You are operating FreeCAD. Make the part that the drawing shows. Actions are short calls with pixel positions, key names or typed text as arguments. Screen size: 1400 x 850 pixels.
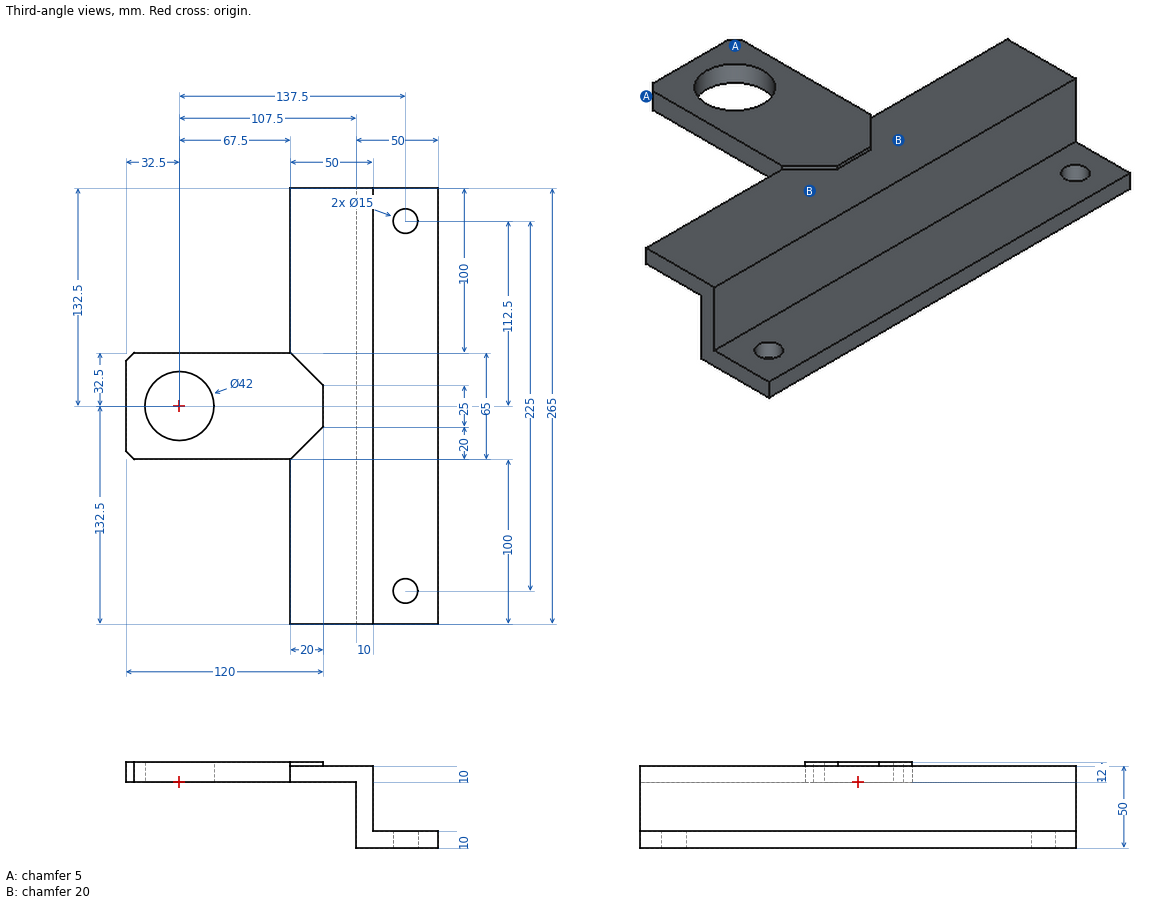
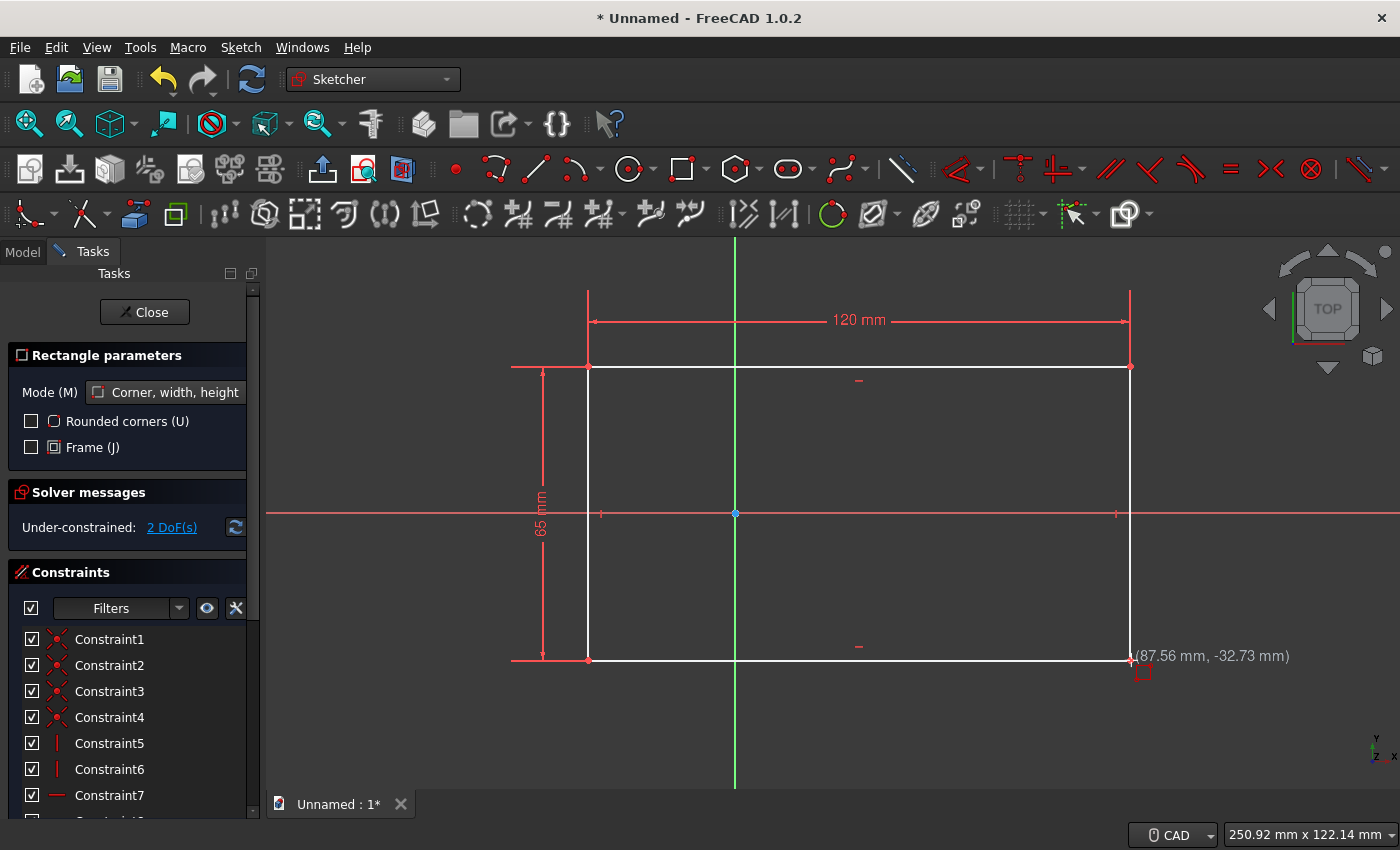
click(630, 170)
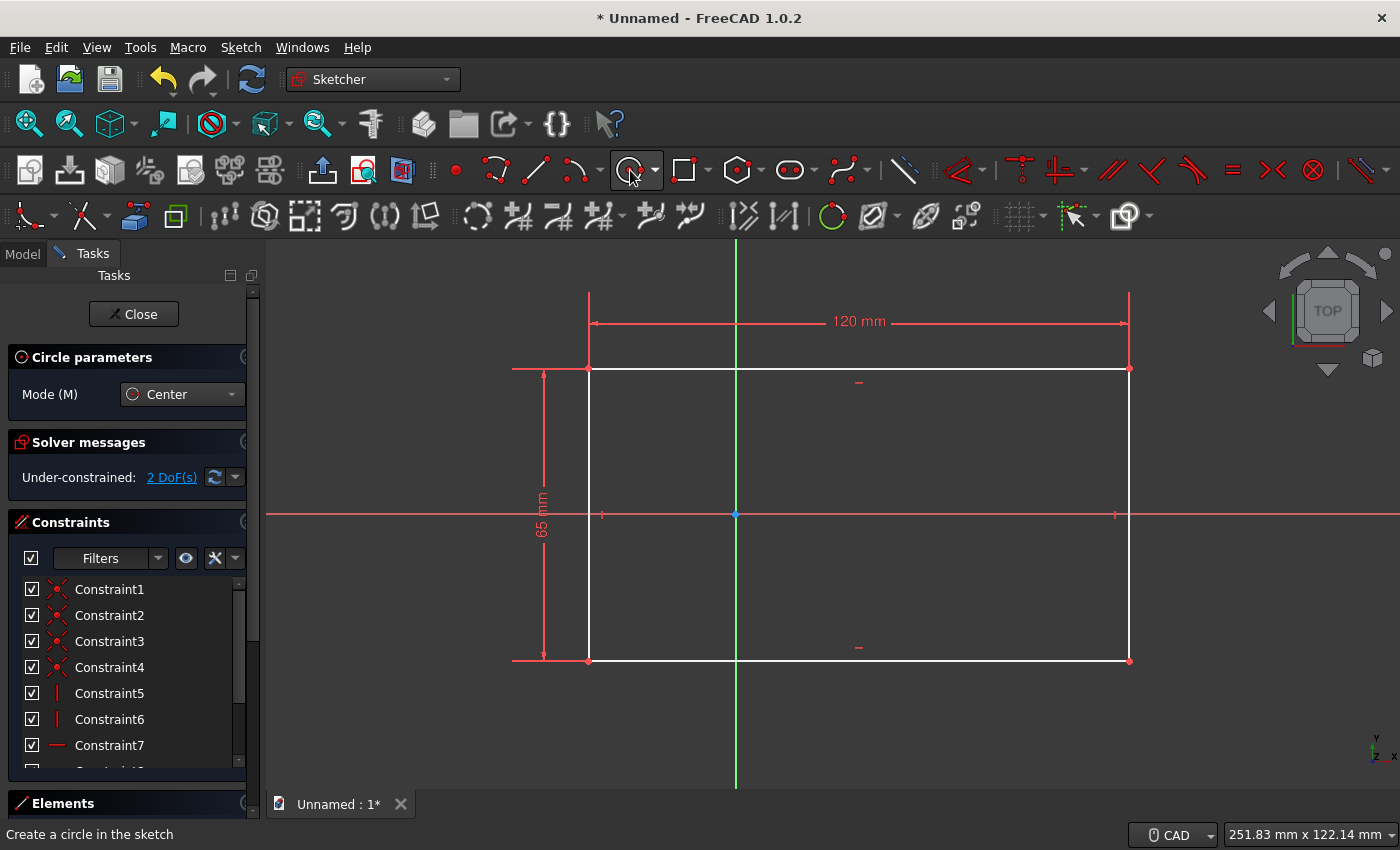
click(736, 514)
move(803, 447)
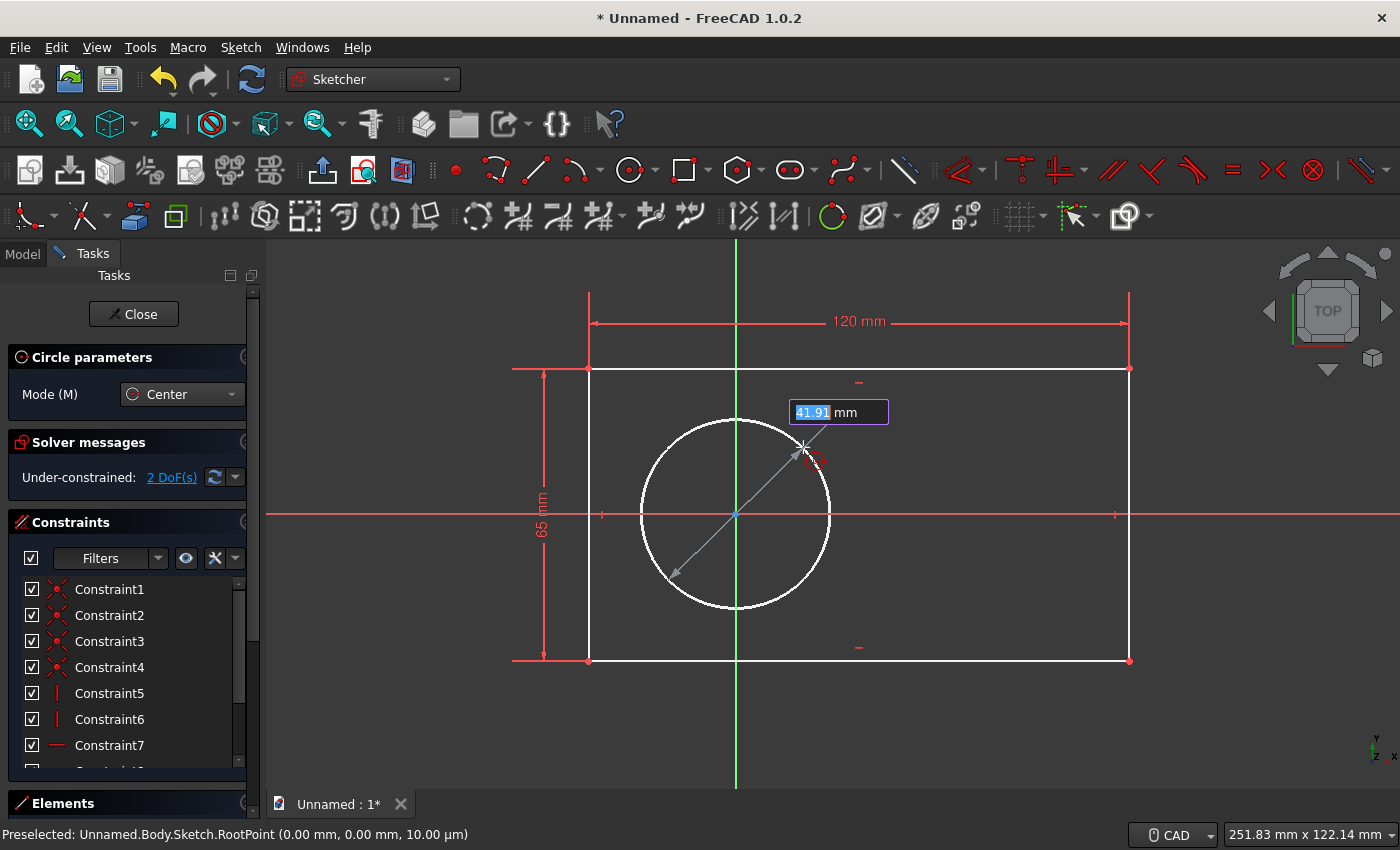
text(42)
key(Return)
key(Escape)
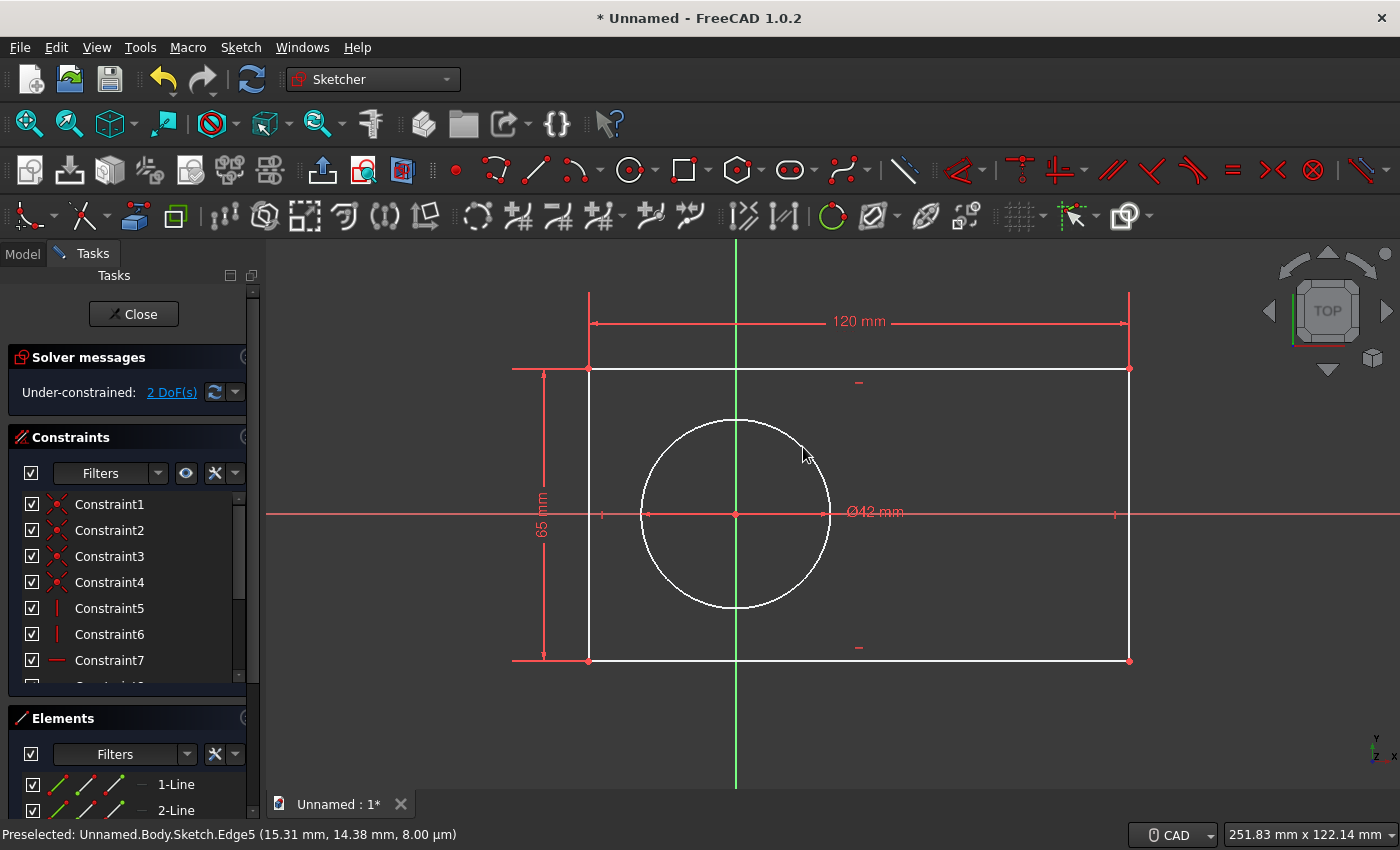
click(589, 369)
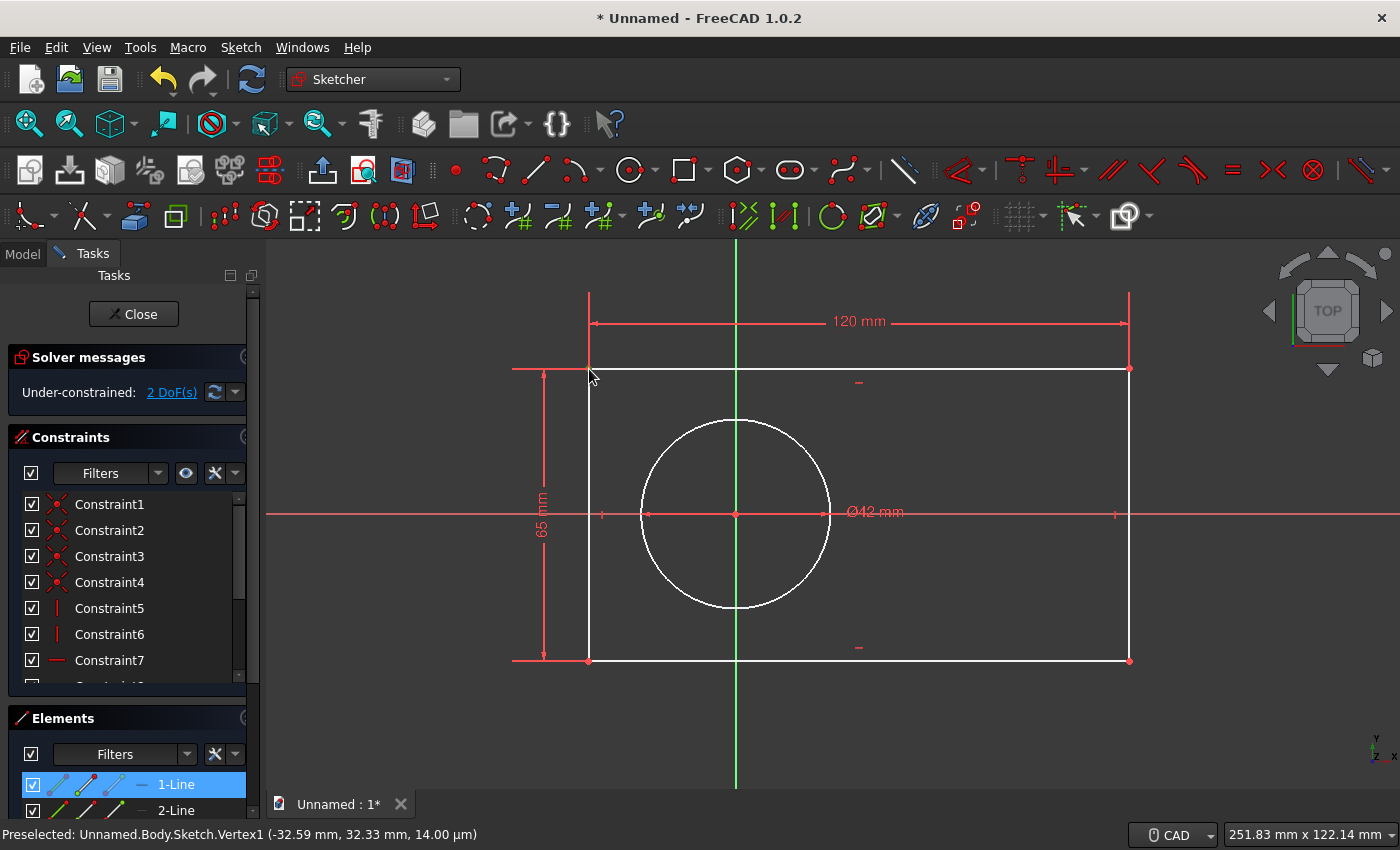
key(l)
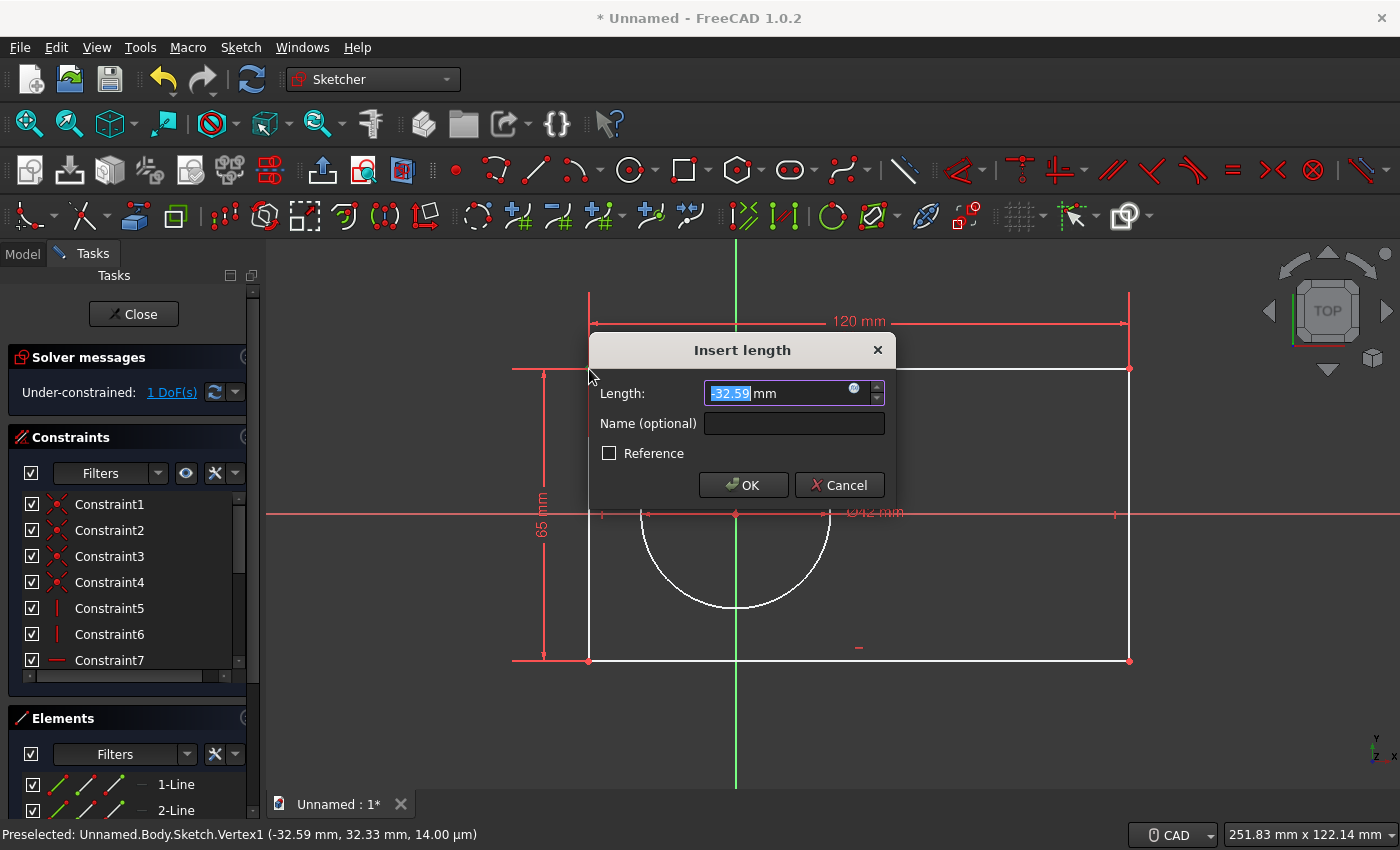
text(-32.5)
key(Return)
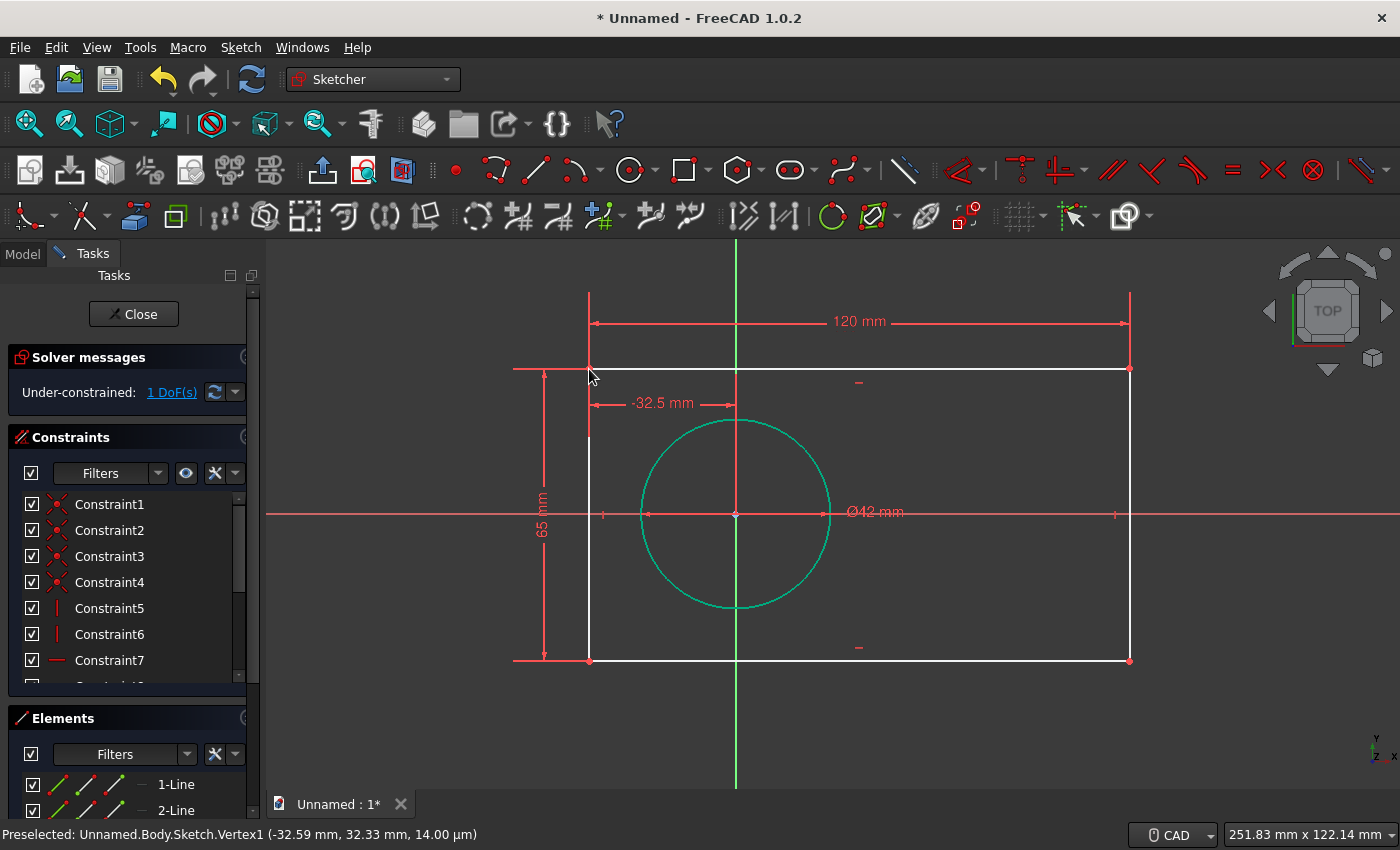
click(589, 369)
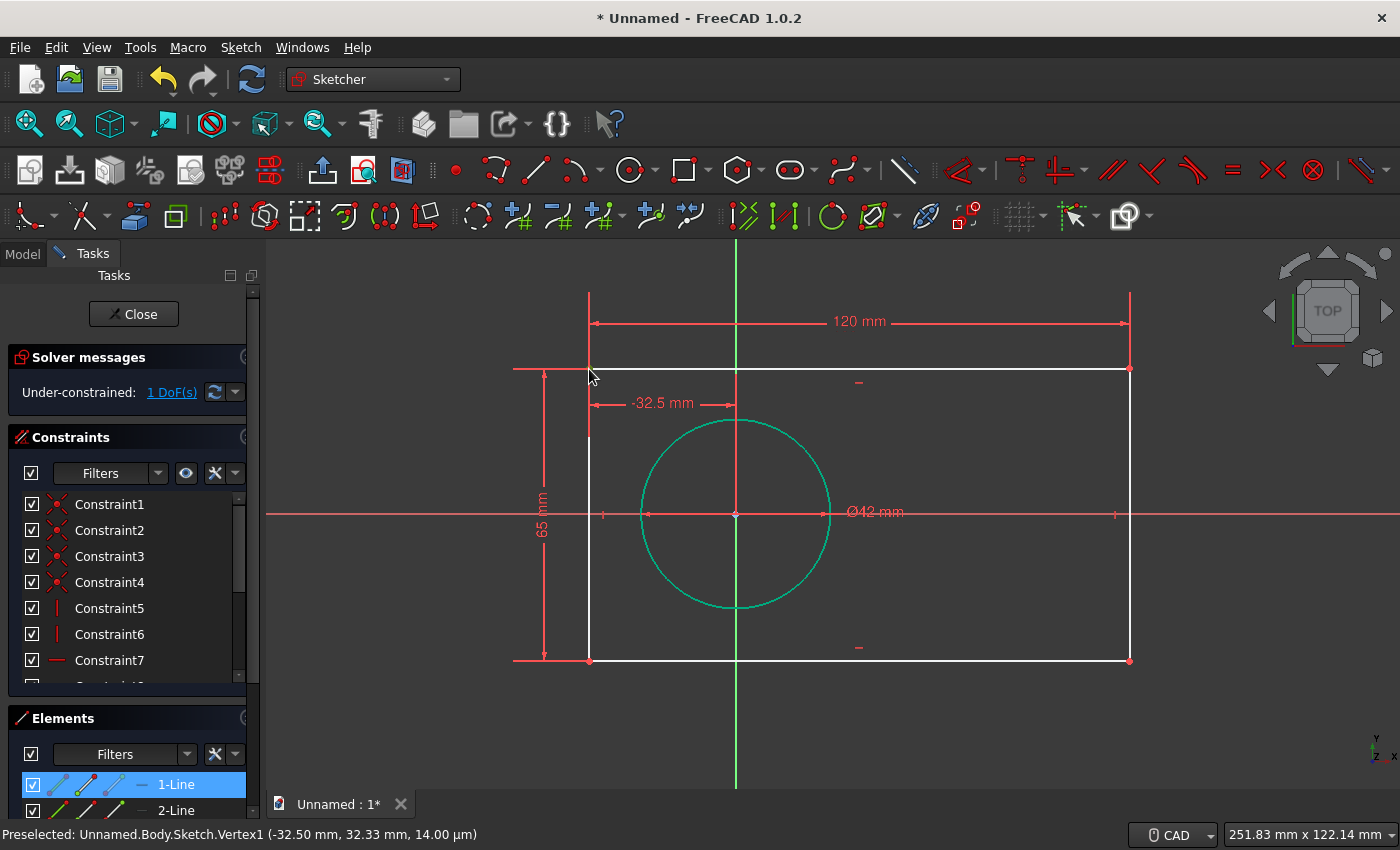
key(i)